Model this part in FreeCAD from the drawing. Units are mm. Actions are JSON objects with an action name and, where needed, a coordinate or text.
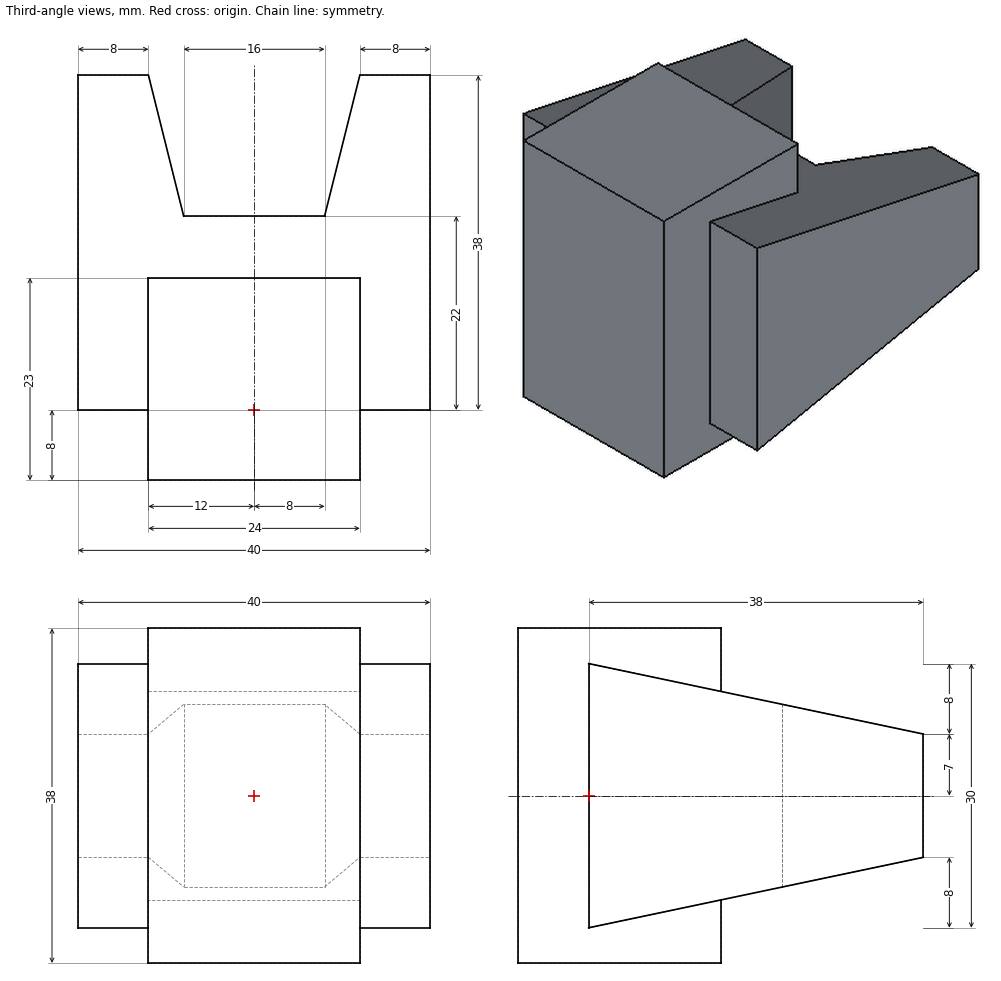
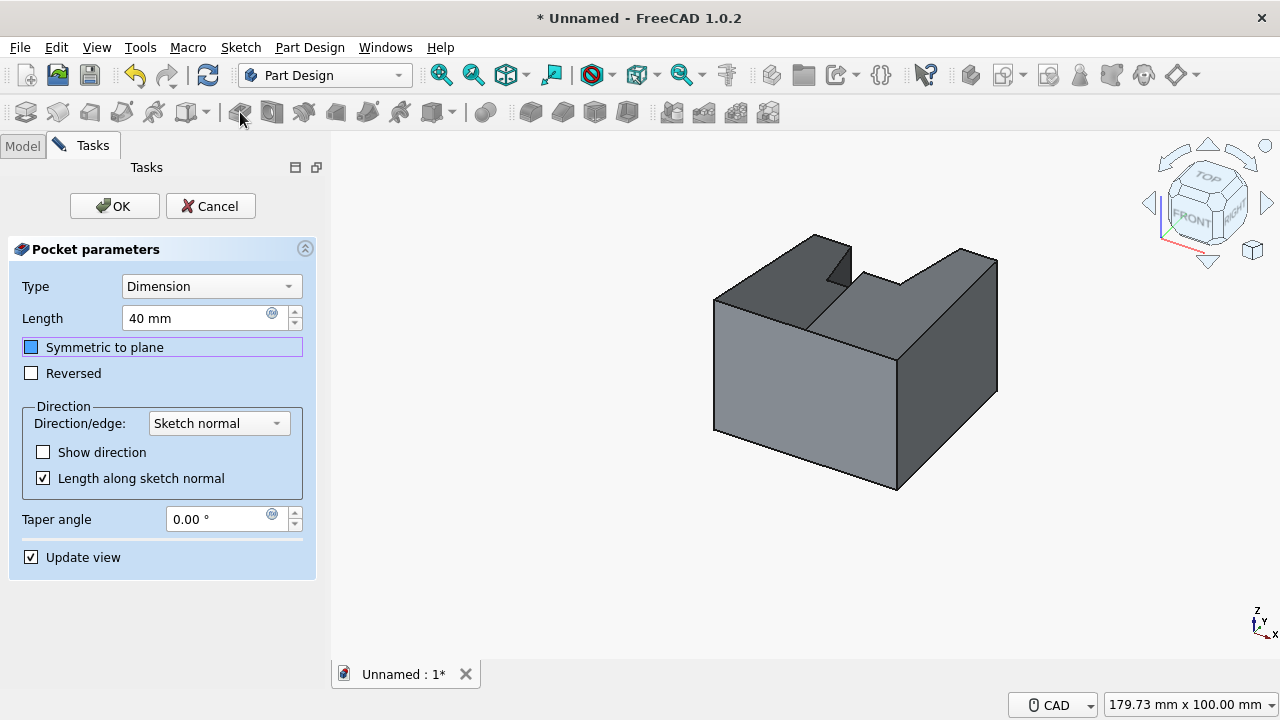
{"action": "left_click", "coordinate": [30, 347]}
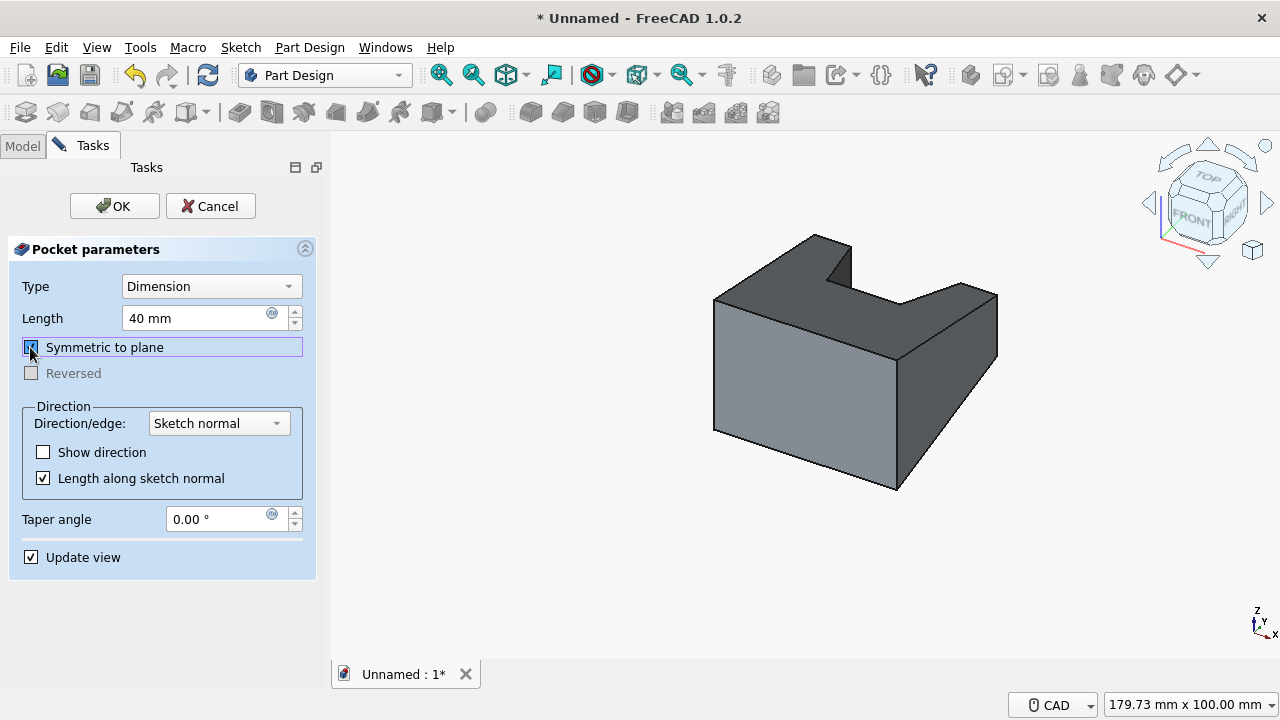
{"action": "left_click", "coordinate": [115, 206]}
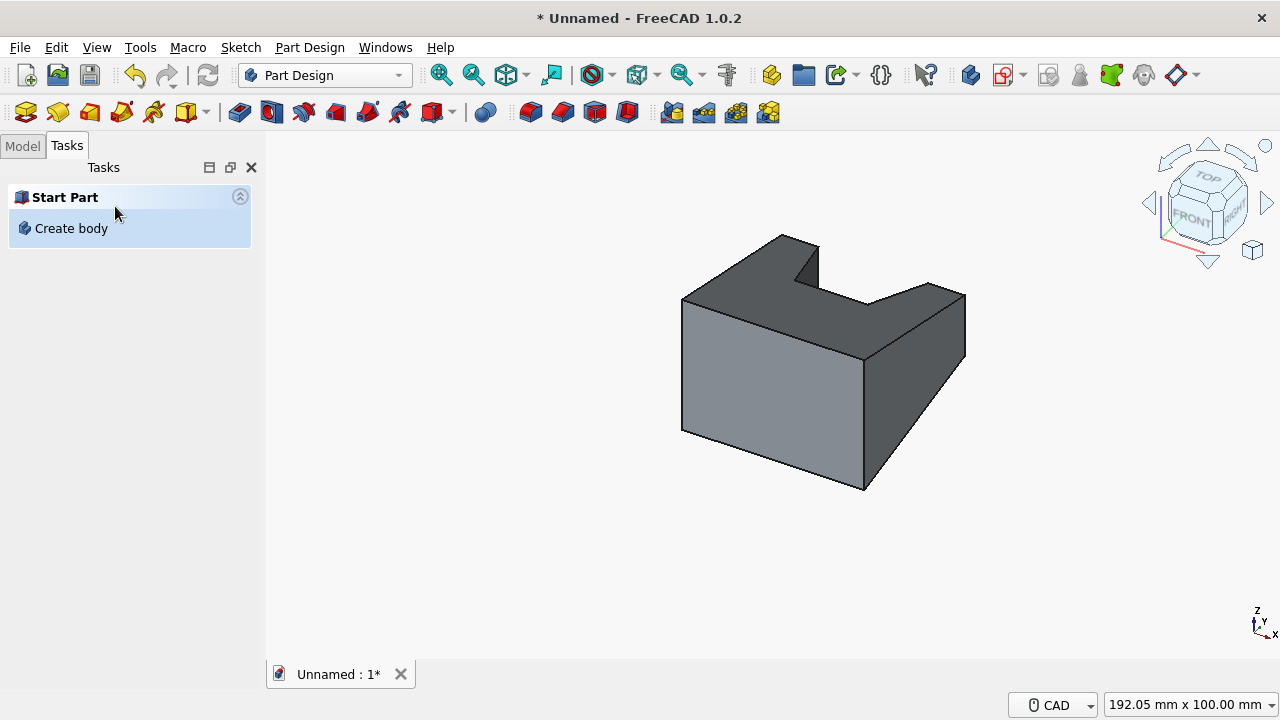
{"action": "left_click", "coordinate": [1004, 76]}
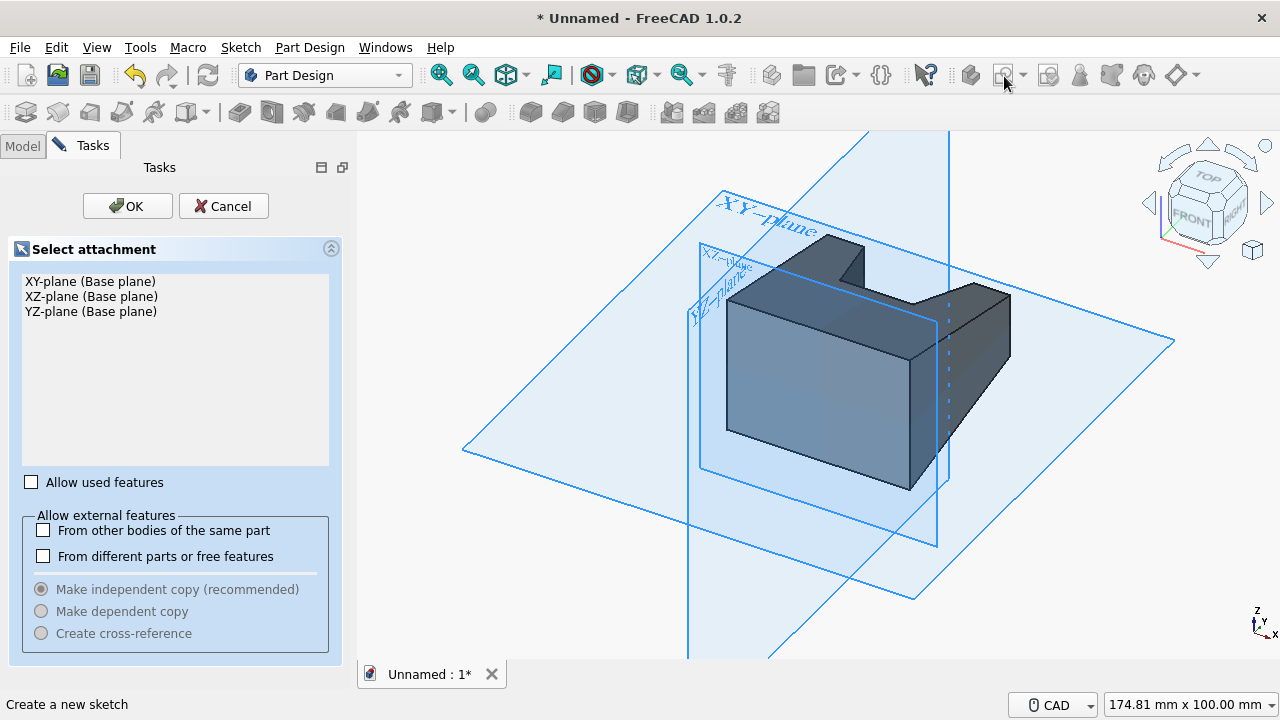
{"action": "left_click", "coordinate": [82, 282]}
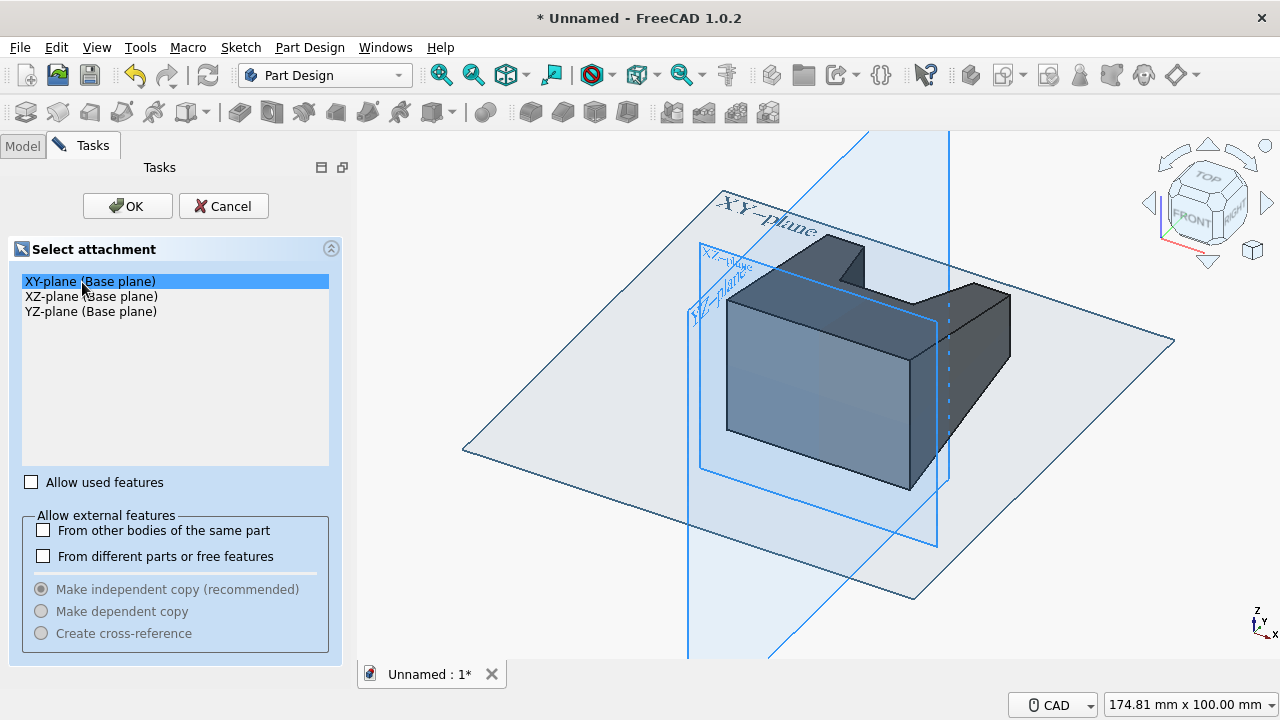
{"action": "left_click", "coordinate": [128, 206]}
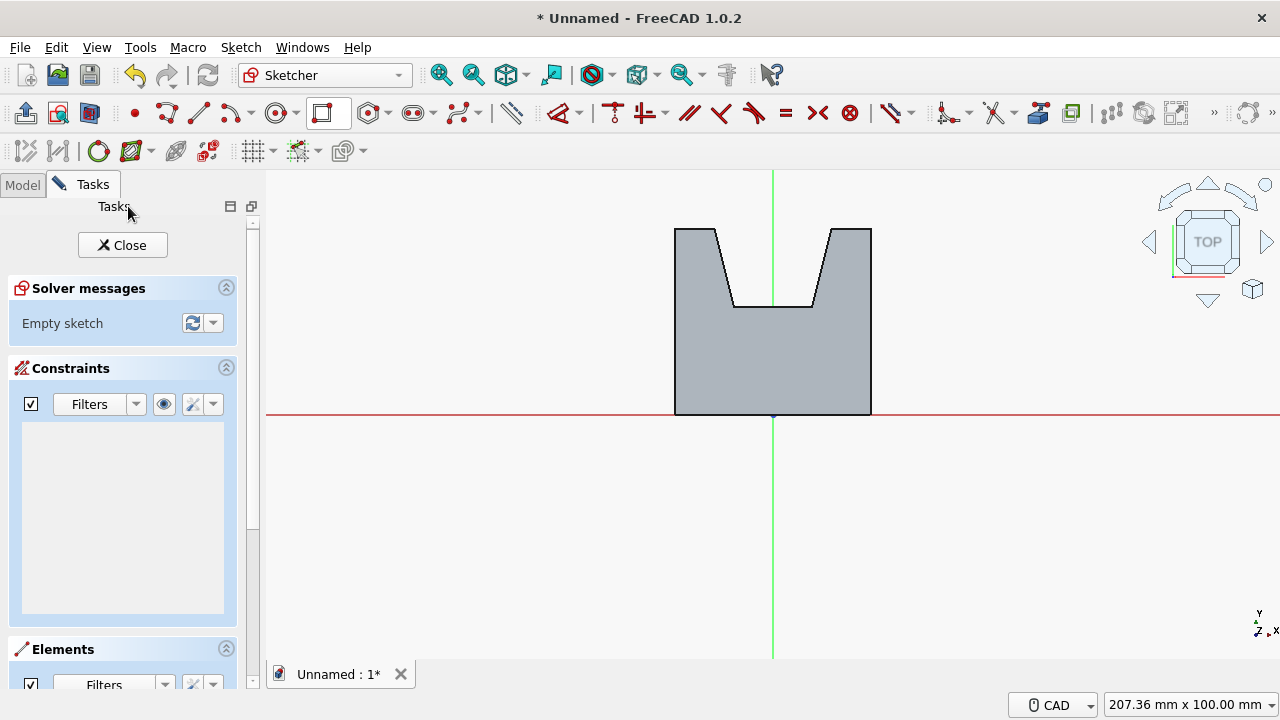
{"action": "left_click", "coordinate": [90, 114]}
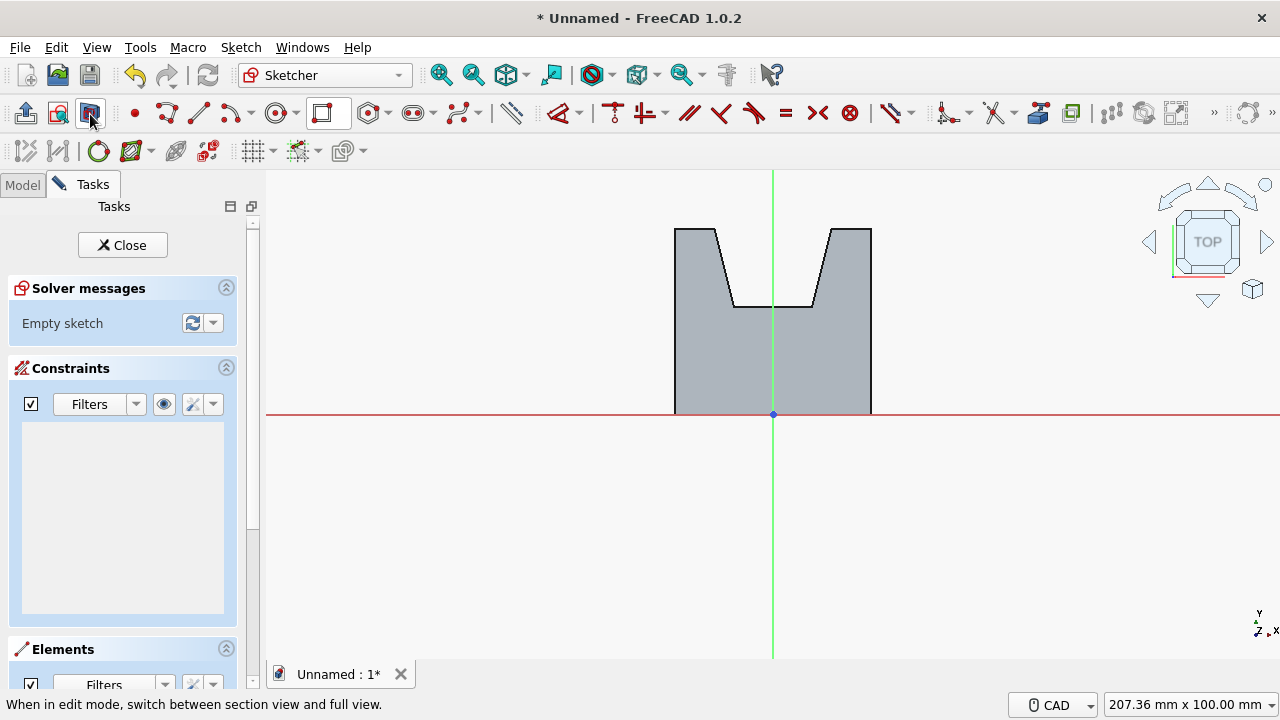
{"action": "scroll", "coordinate": [813, 387], "scroll_direction": "up", "scroll_amount": 5}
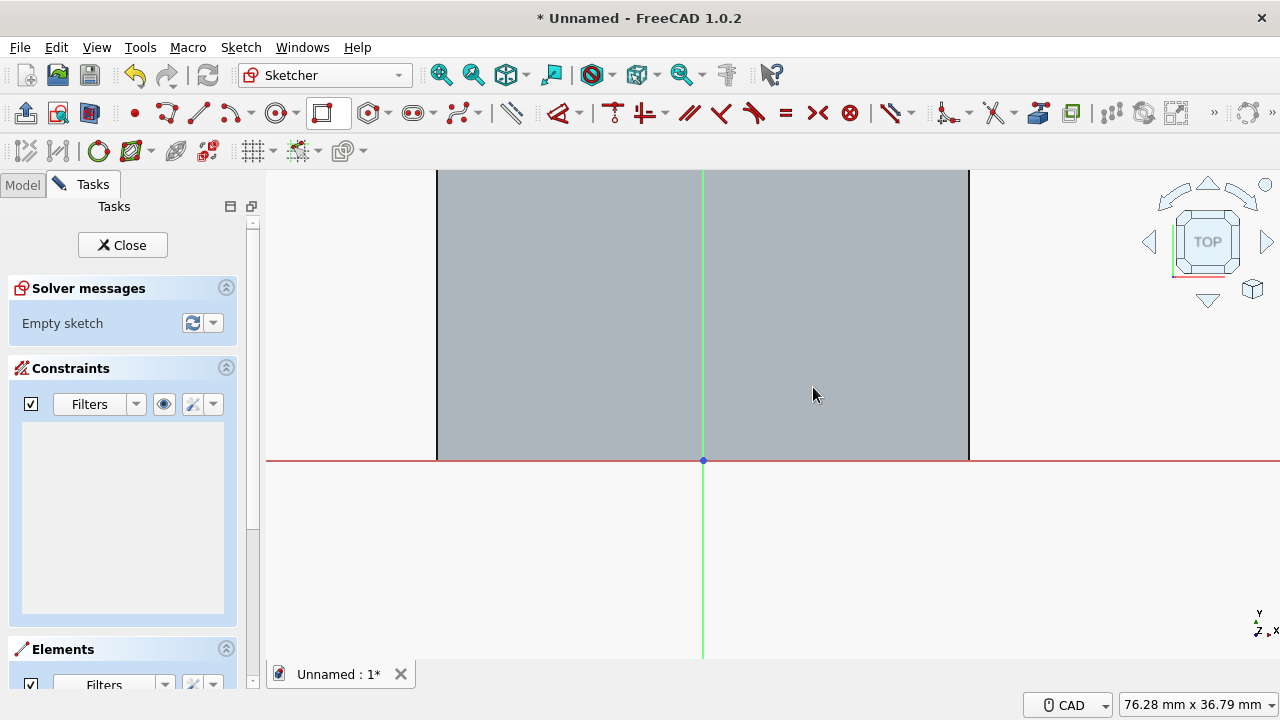
{"action": "left_click", "coordinate": [322, 114]}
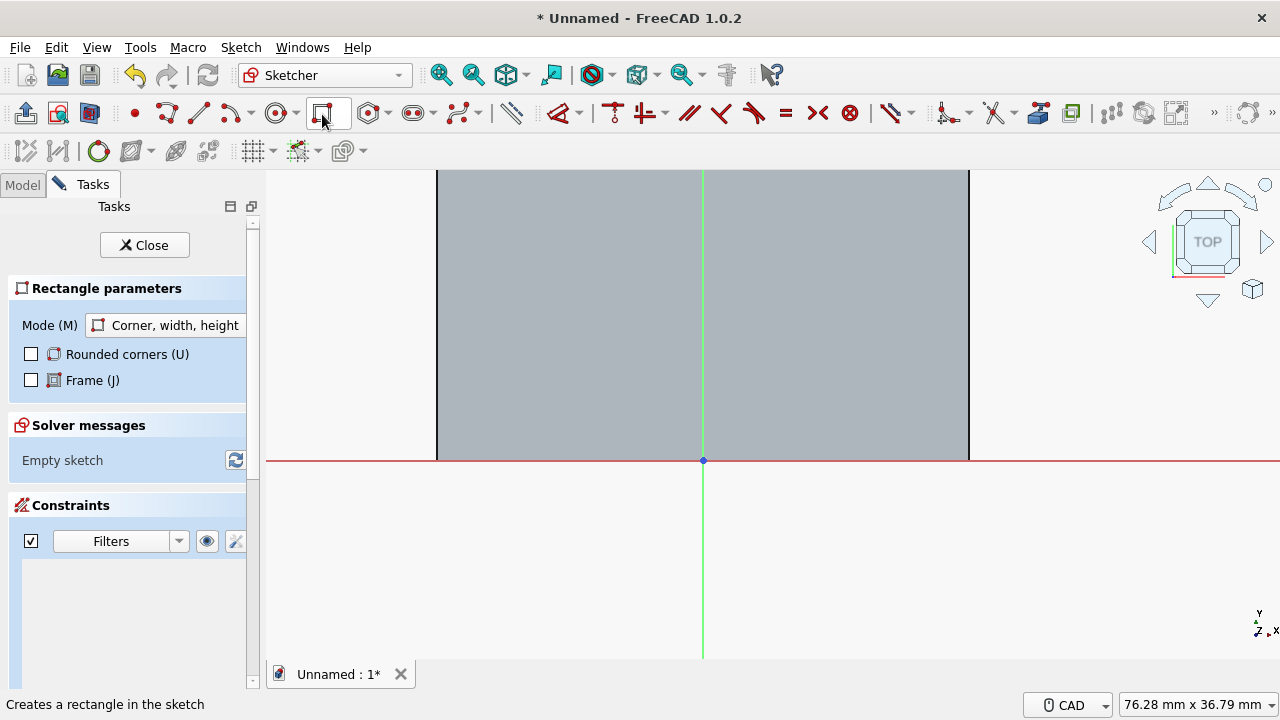
{"action": "left_click", "coordinate": [544, 262]}
{"action": "left_click", "coordinate": [863, 567]}
{"action": "key", "text": "Escape"}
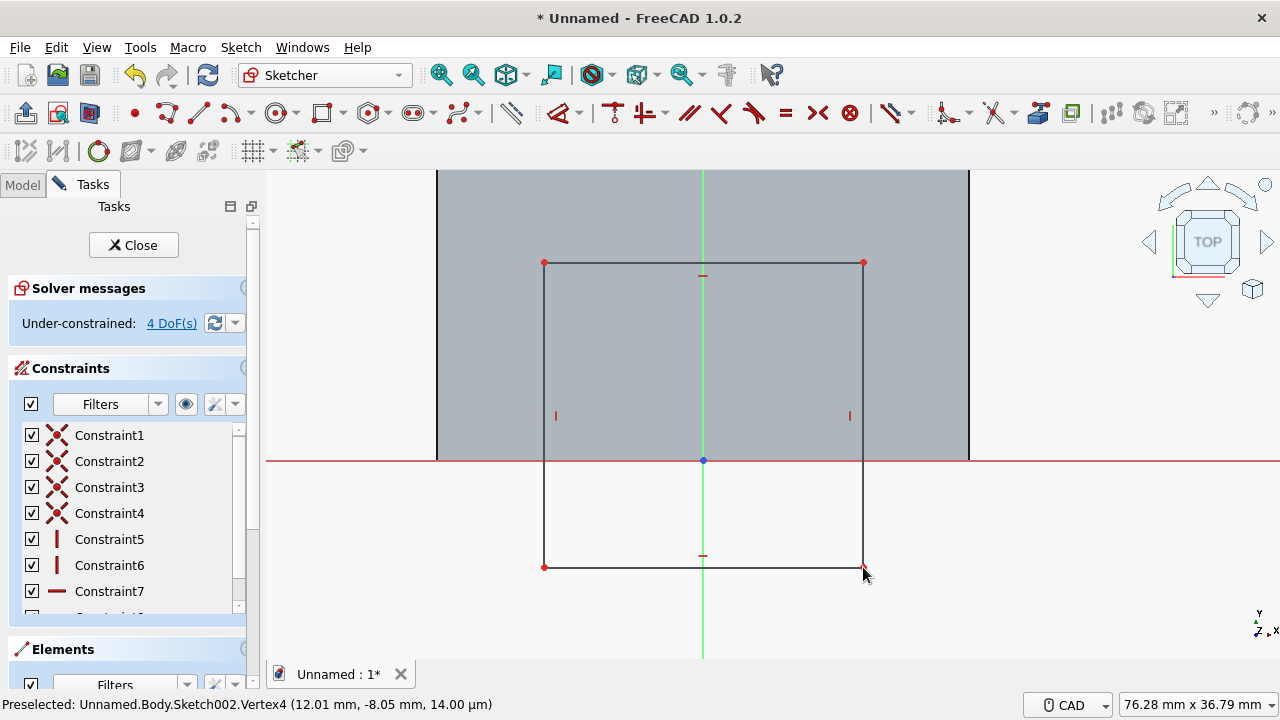
{"action": "left_click", "coordinate": [558, 114]}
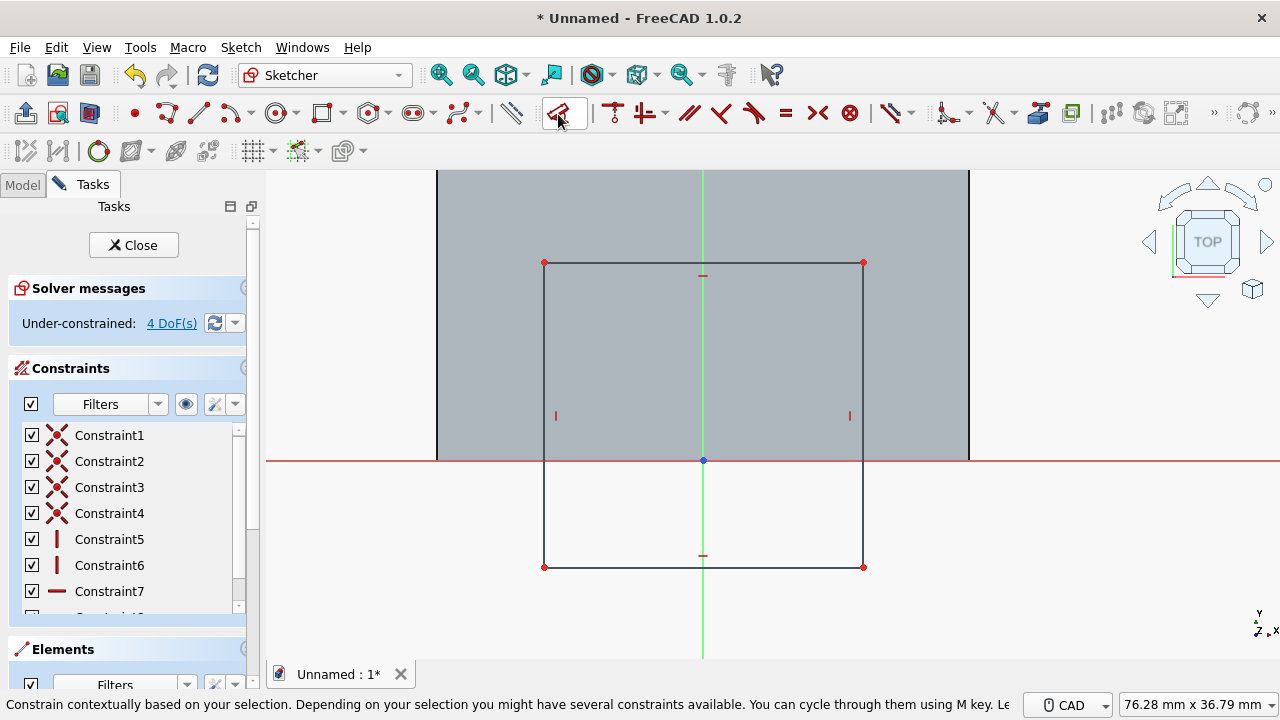
{"action": "left_click", "coordinate": [544, 355]}
{"action": "left_click", "coordinate": [510, 416]}